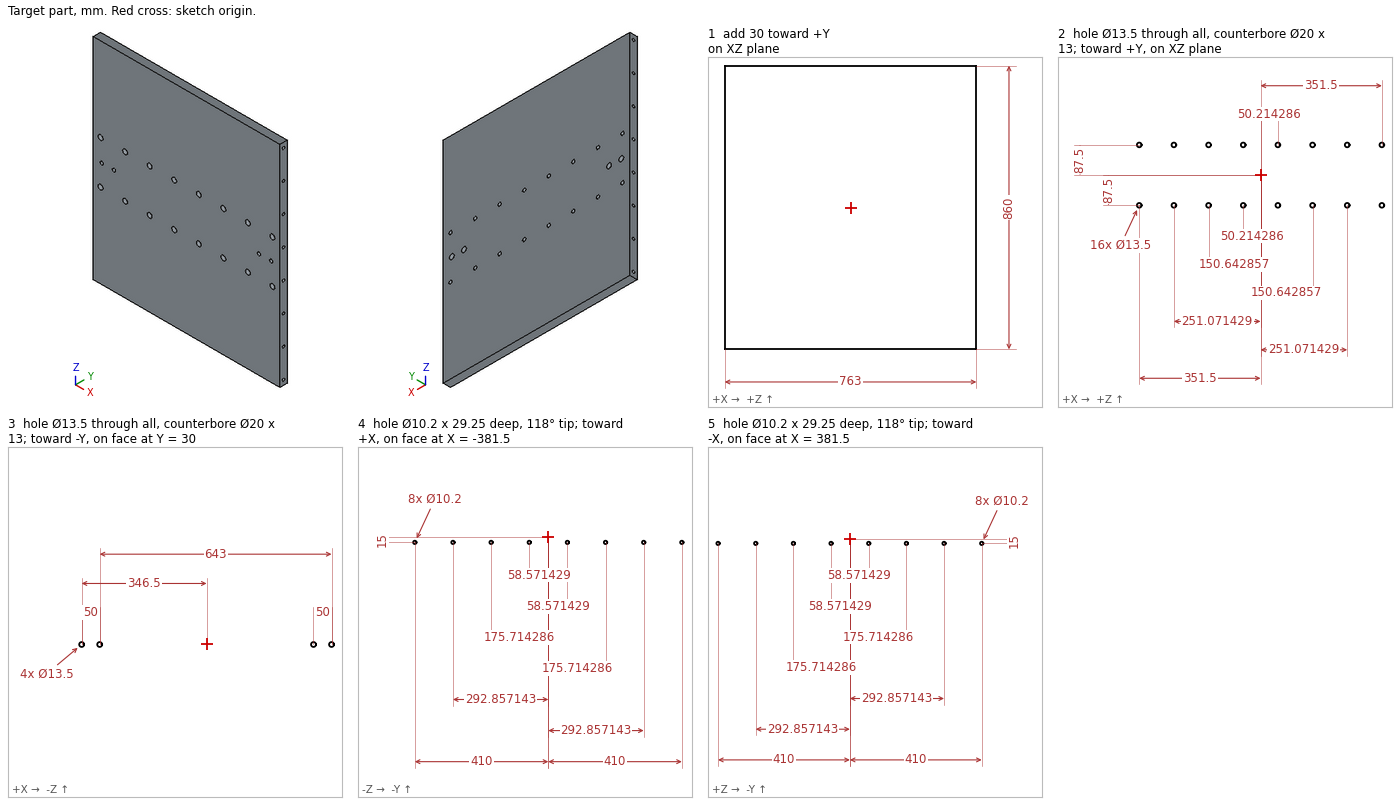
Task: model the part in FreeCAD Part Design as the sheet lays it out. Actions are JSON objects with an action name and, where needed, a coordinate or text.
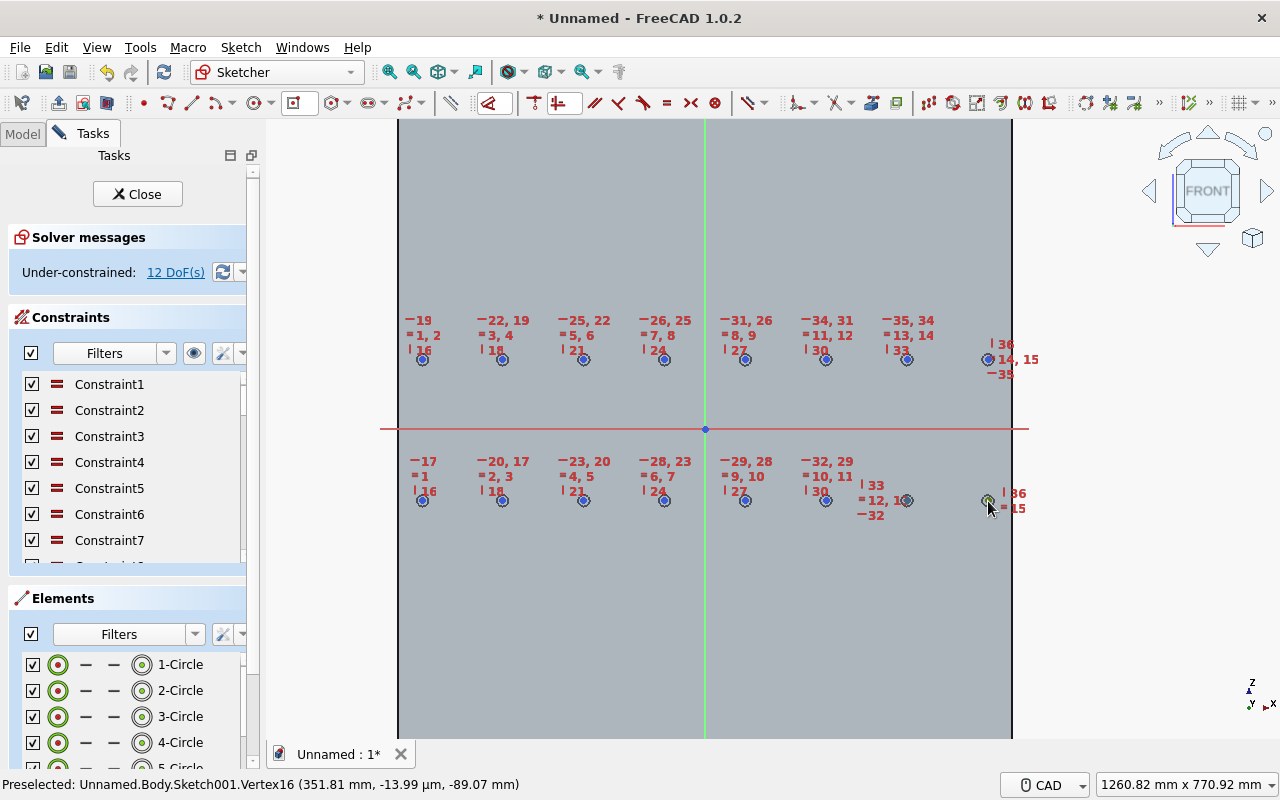
{"action": "key", "text": "h"}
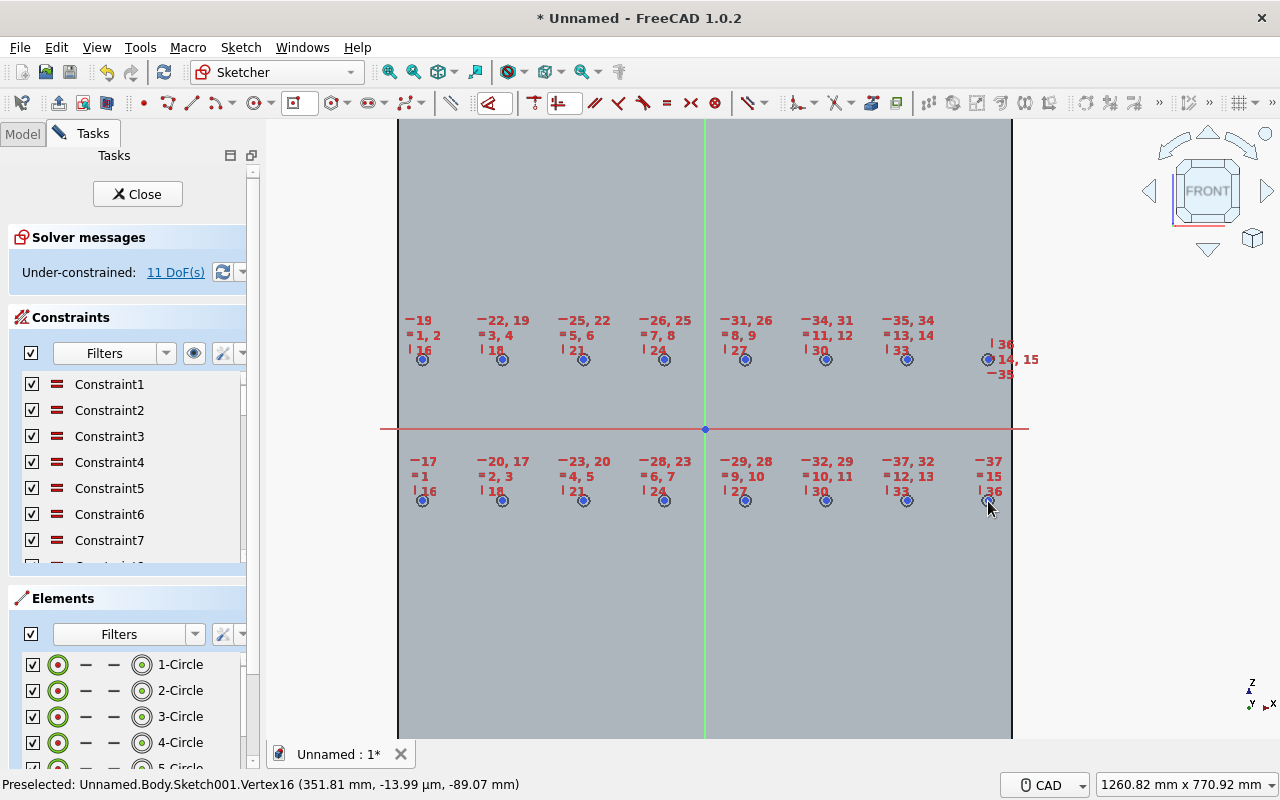
{"action": "scroll", "coordinate": [419, 505], "scroll_direction": "up", "scroll_amount": 7}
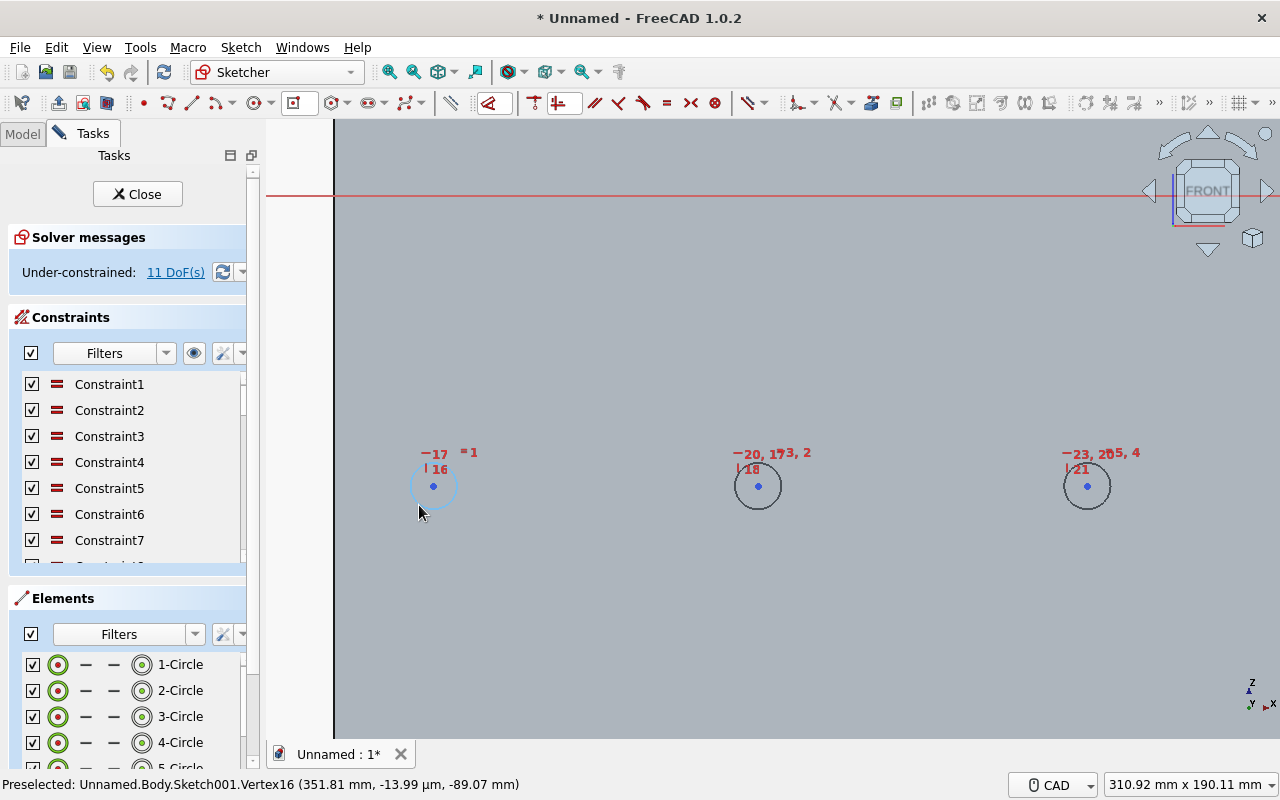
{"action": "left_click", "coordinate": [417, 503]}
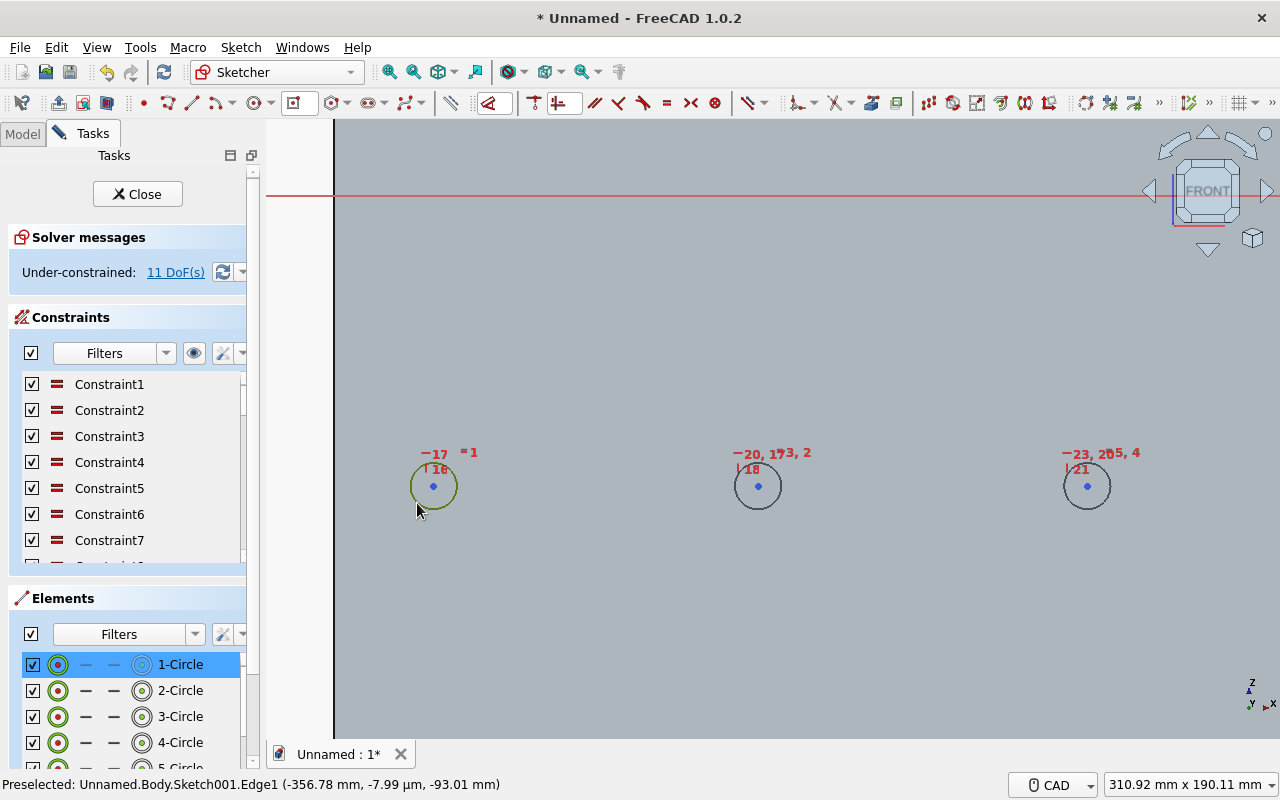
{"action": "left_click", "coordinate": [506, 104]}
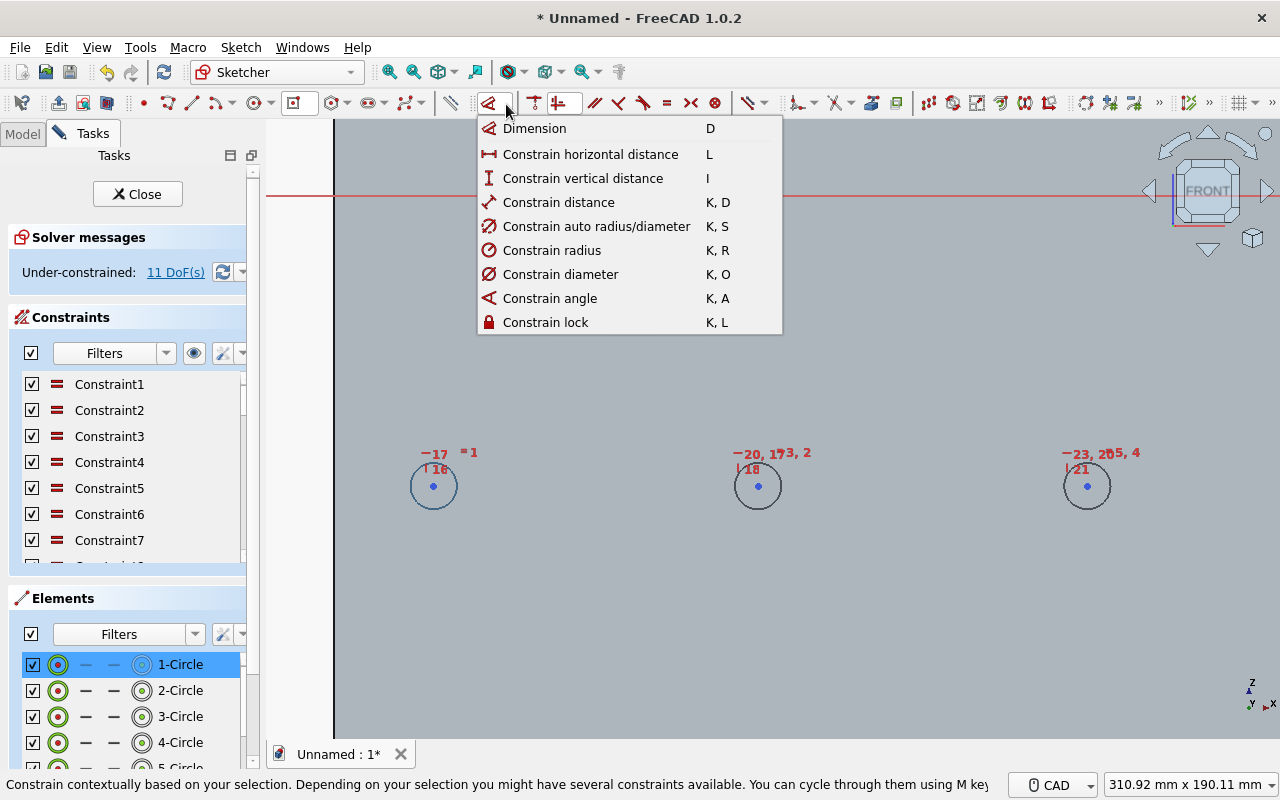
{"action": "left_click", "coordinate": [630, 274]}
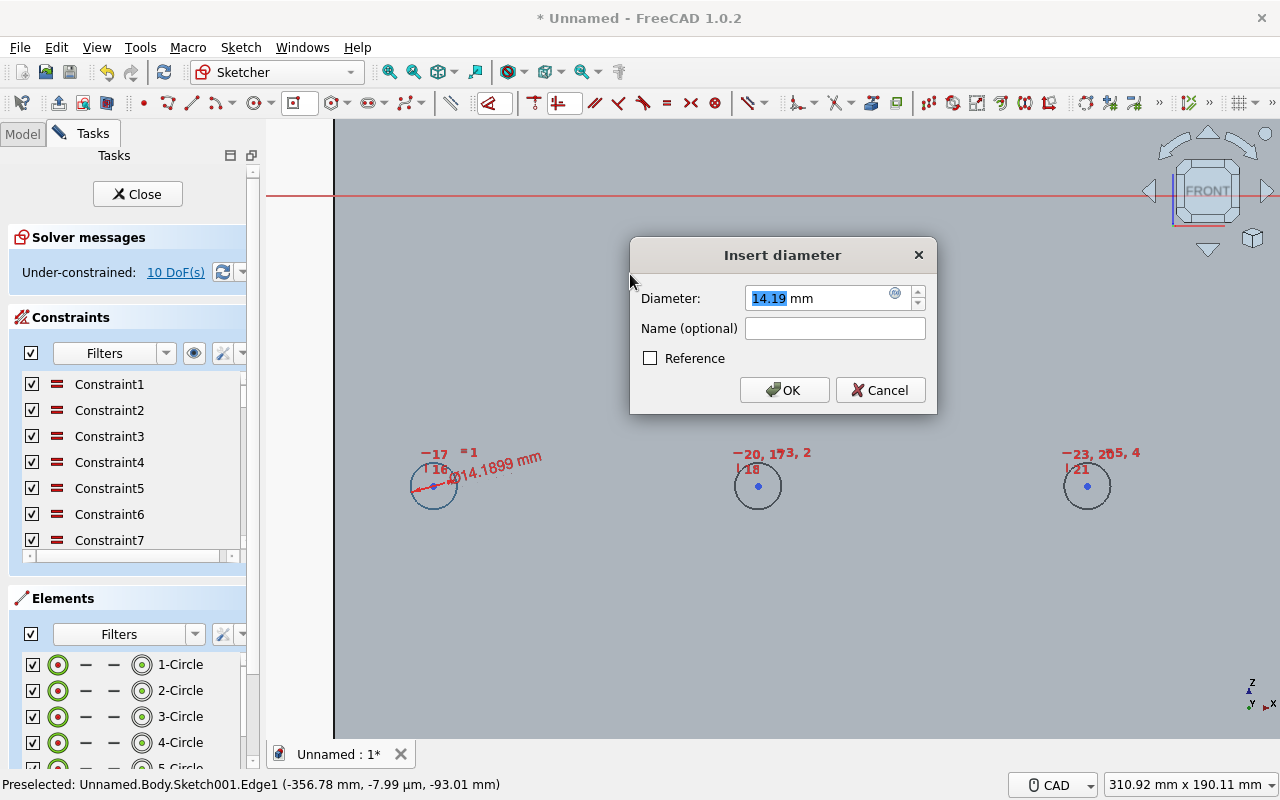
{"action": "type", "text": "13.5"}
{"action": "key", "text": "Return"}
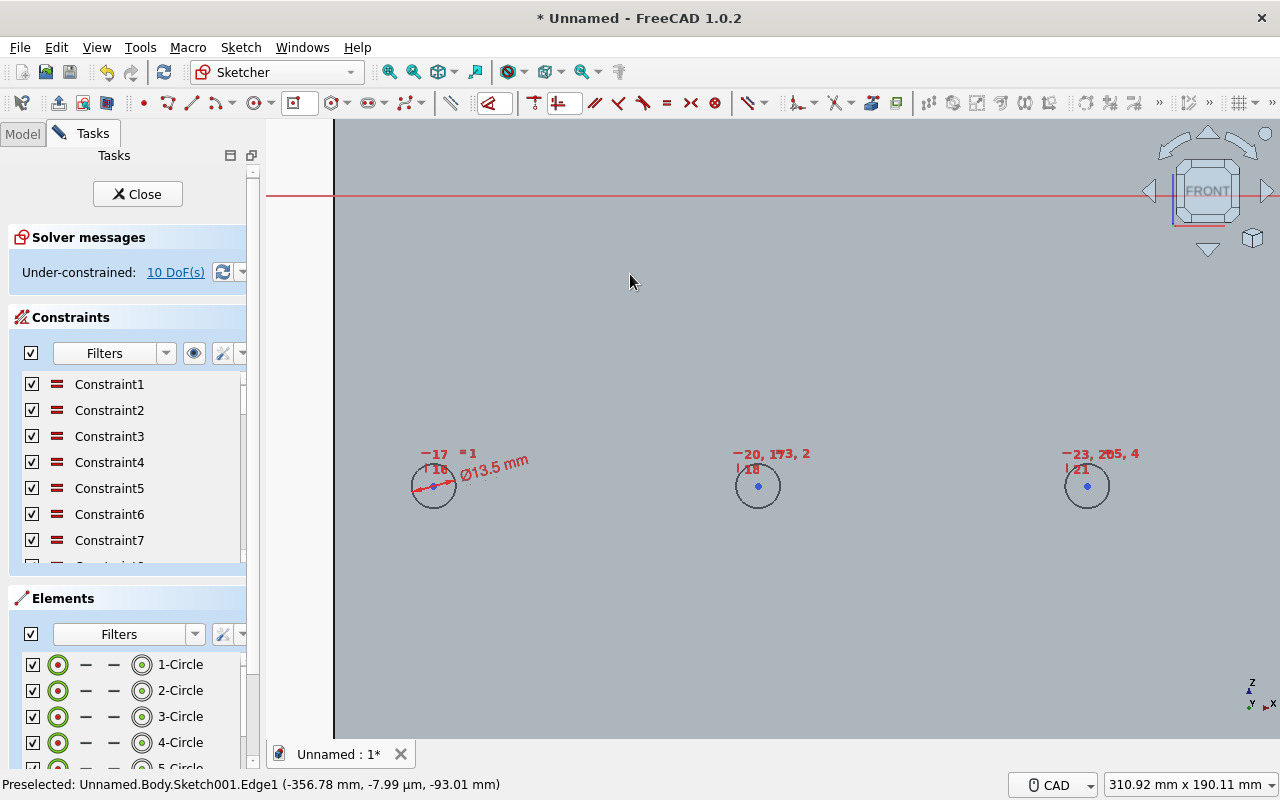
{"action": "scroll", "coordinate": [418, 505], "scroll_direction": "down", "scroll_amount": 7}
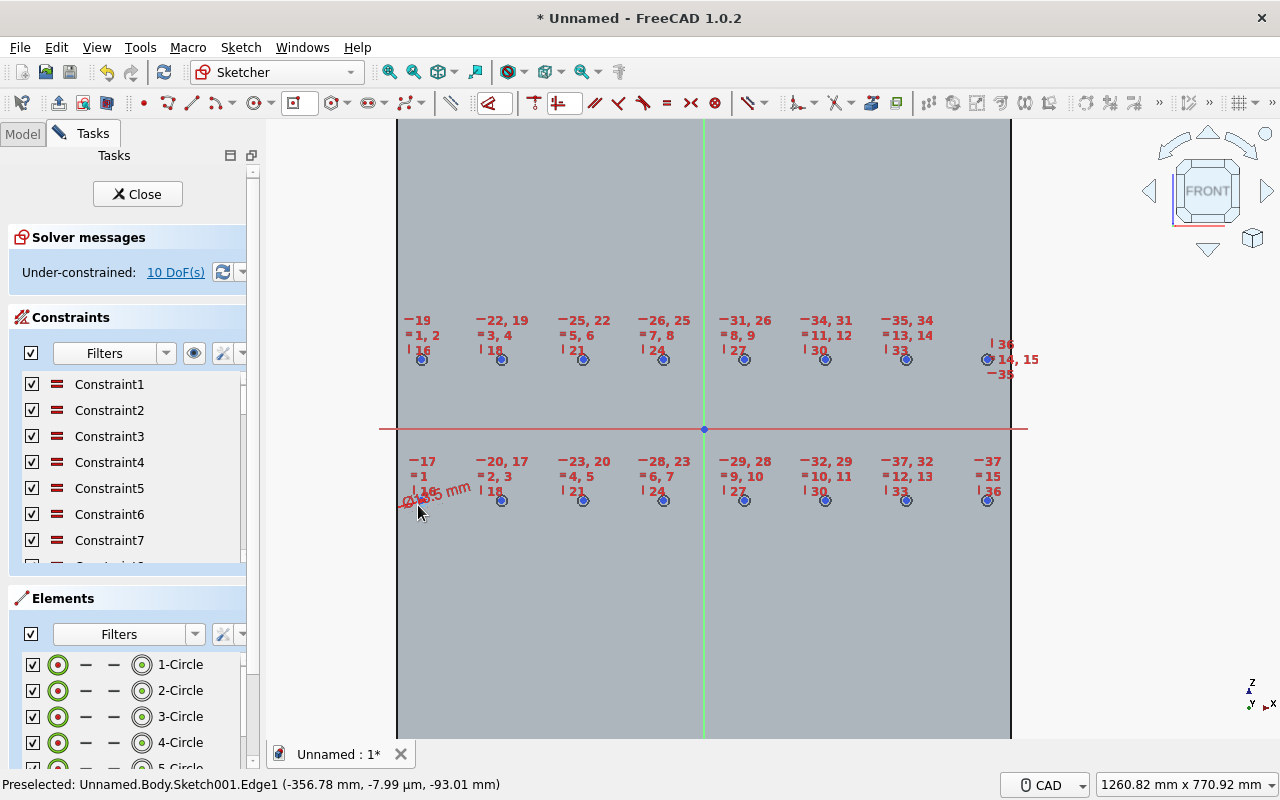
{"action": "left_click", "coordinate": [422, 501]}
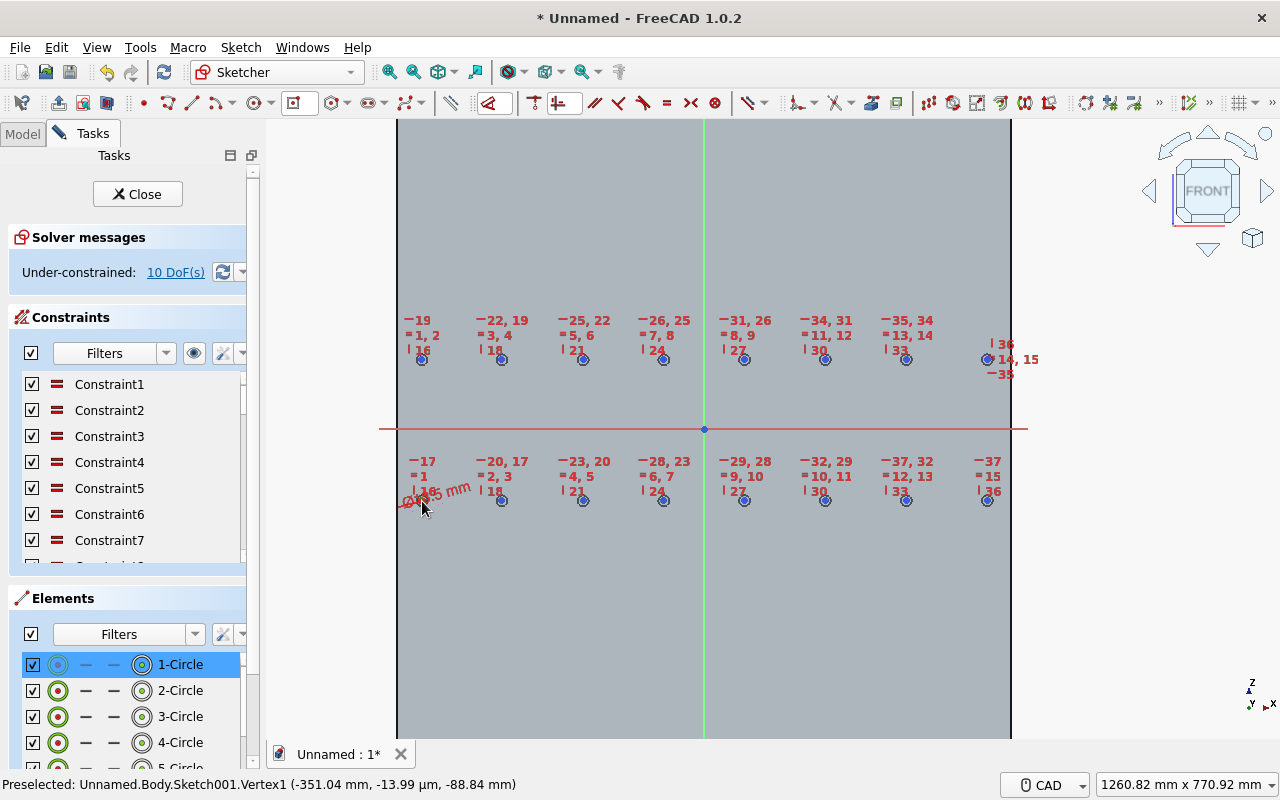
{"action": "left_click", "coordinate": [506, 104]}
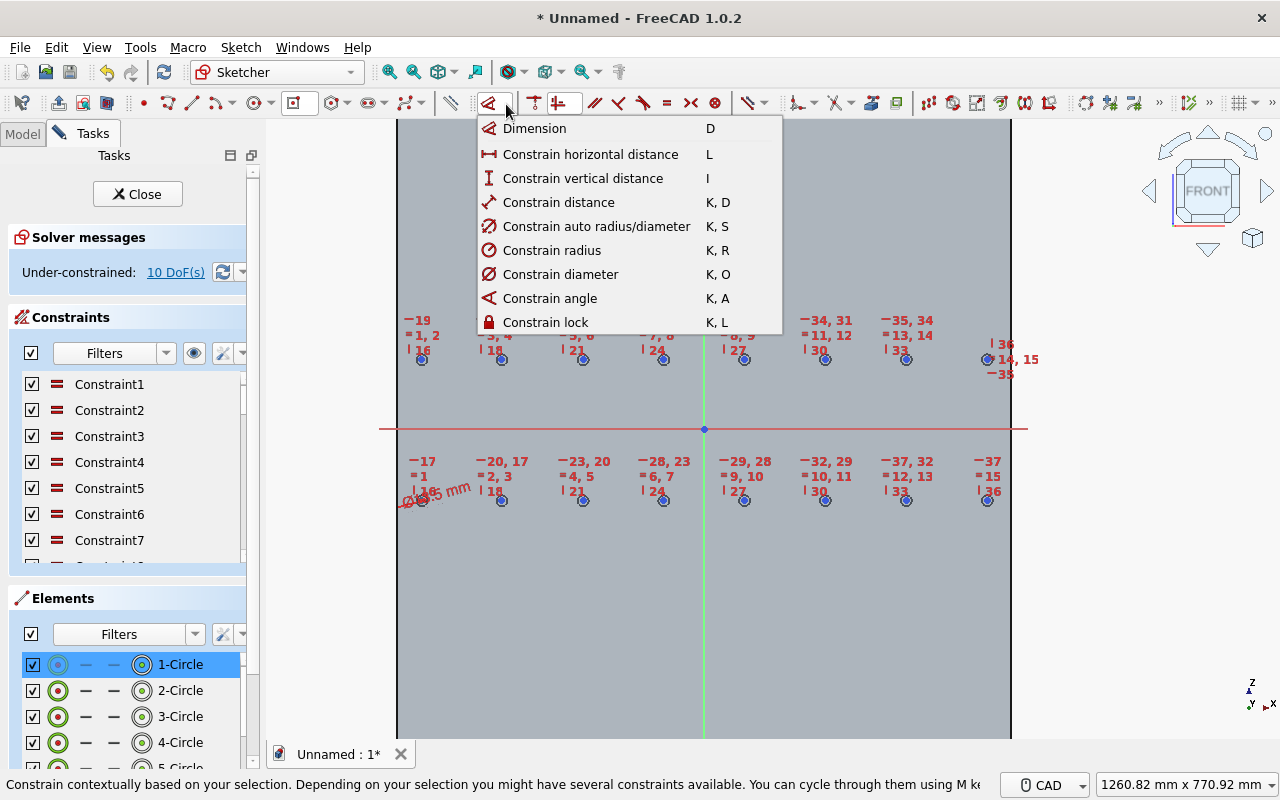
{"action": "left_click", "coordinate": [630, 178]}